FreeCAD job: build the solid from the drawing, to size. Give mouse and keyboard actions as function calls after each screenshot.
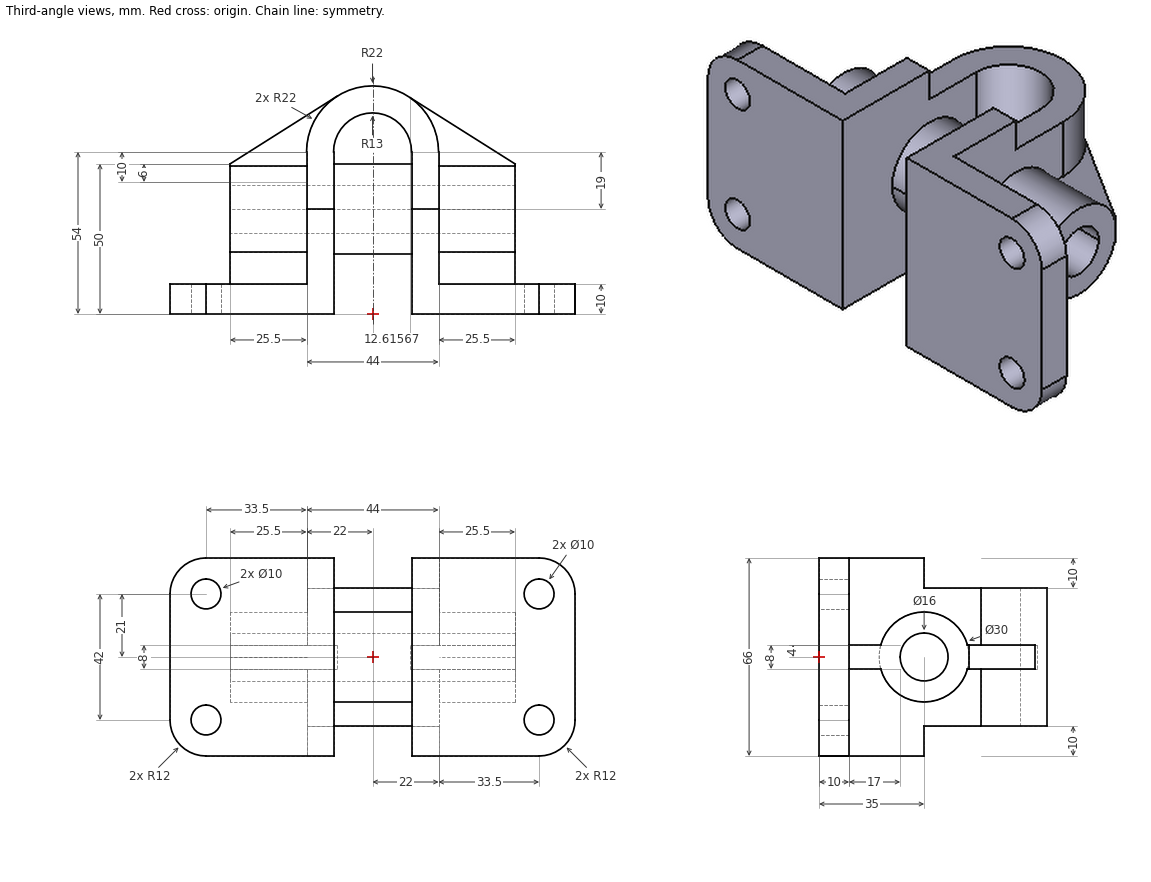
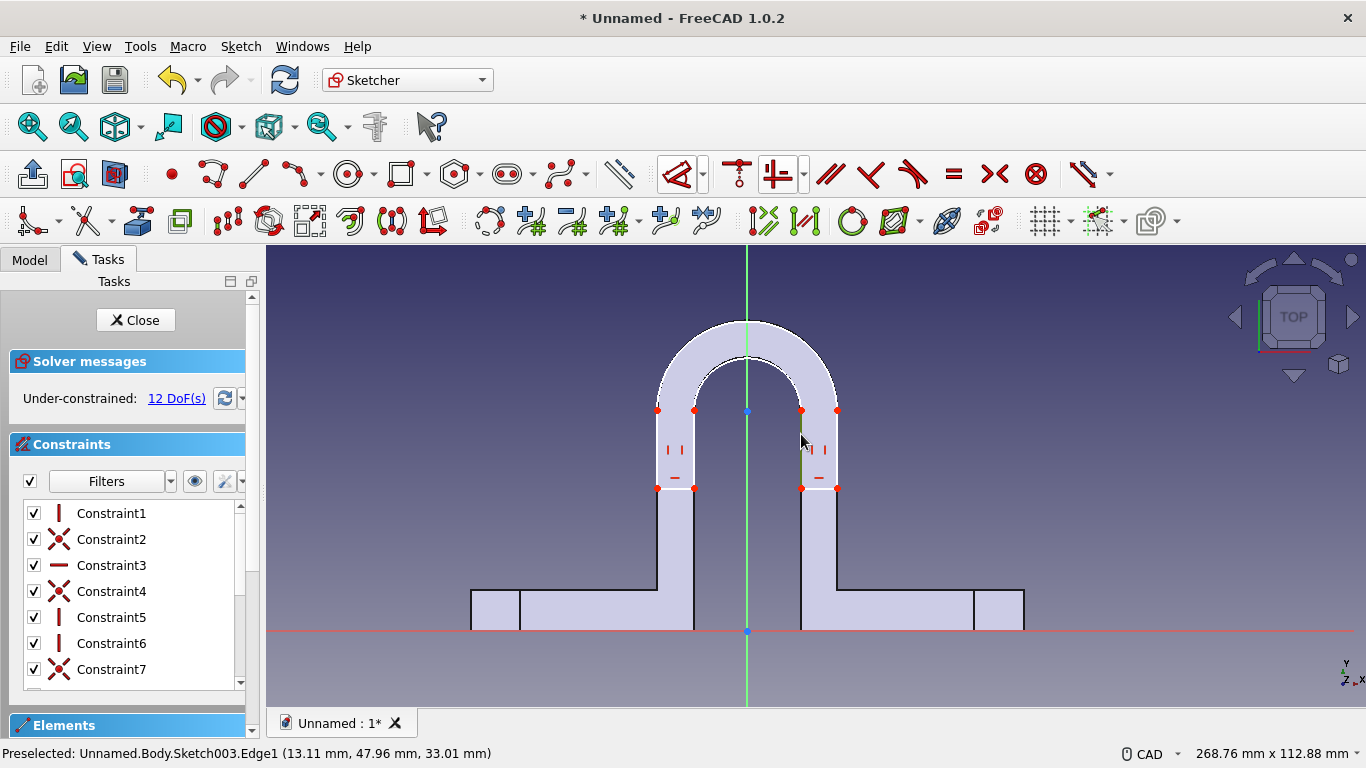
click(779, 368)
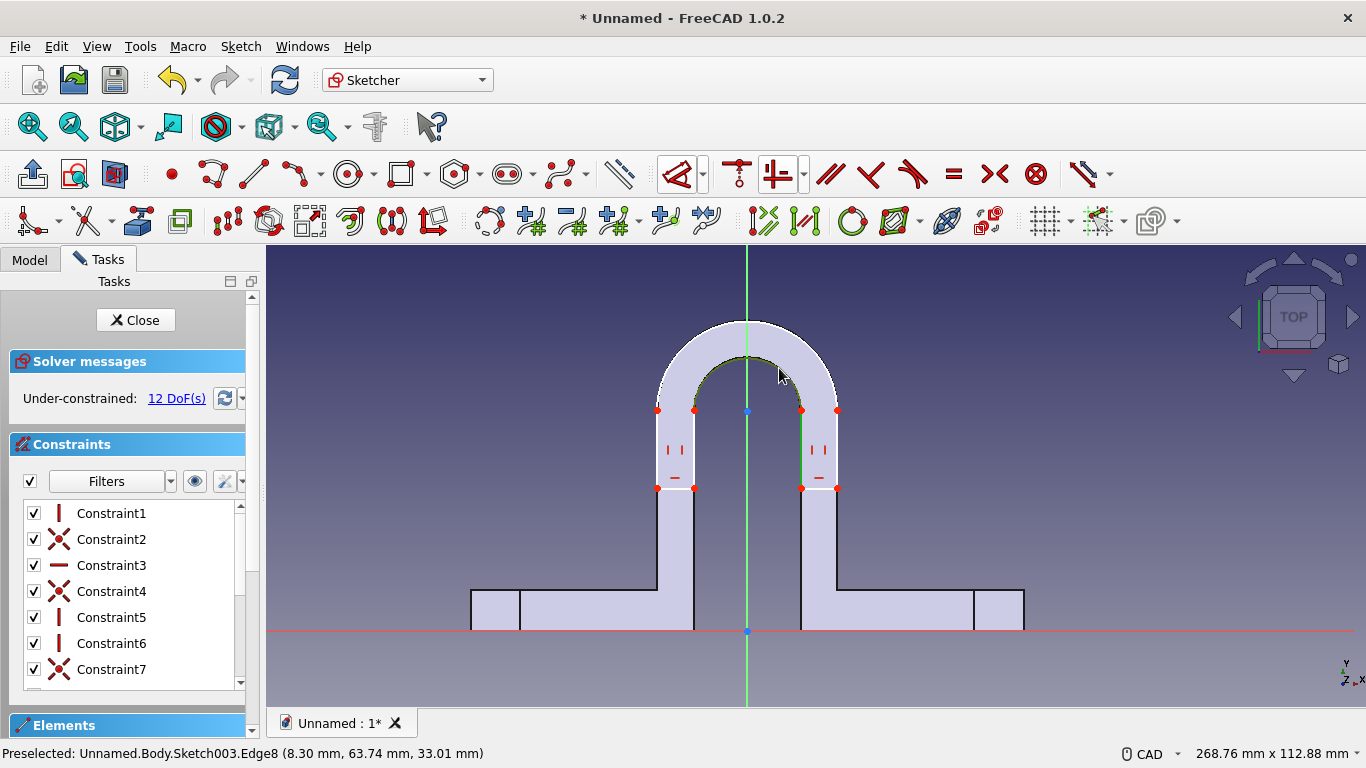
click(913, 174)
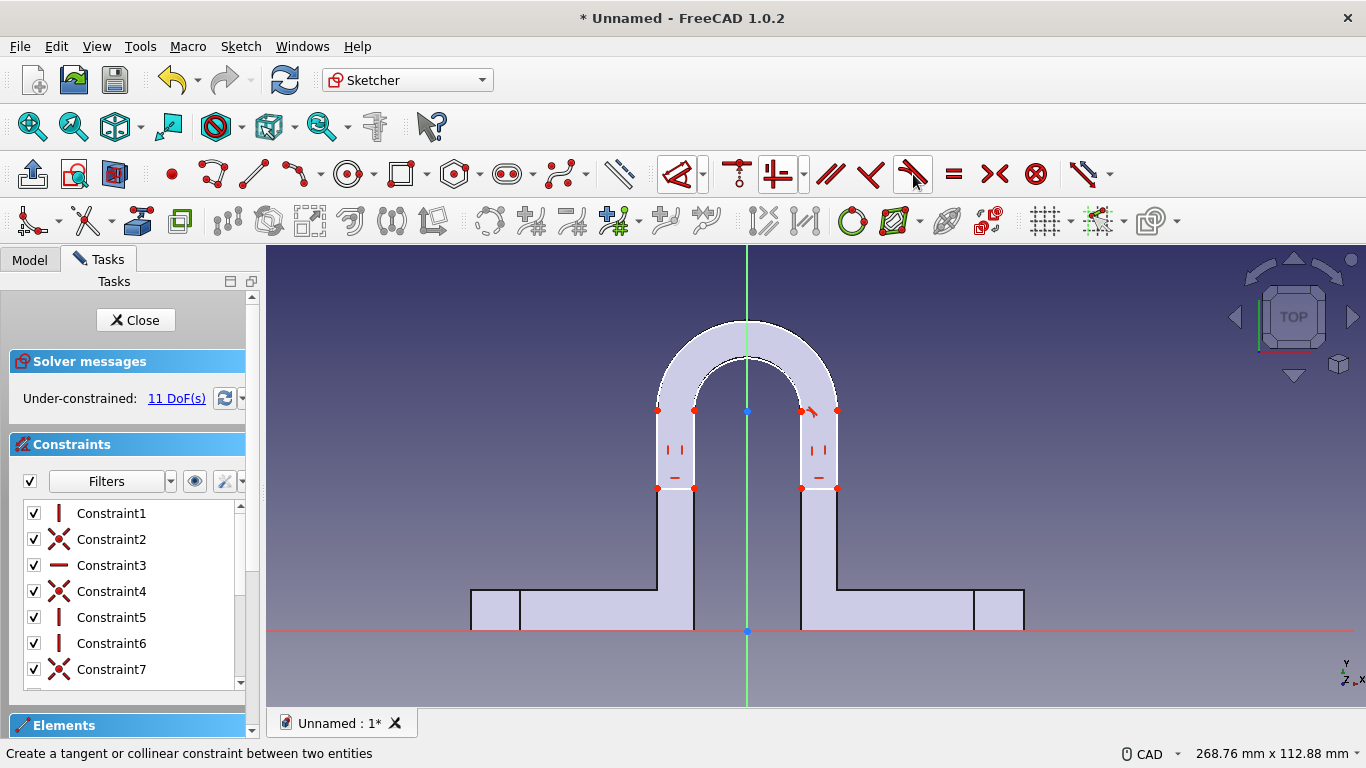
click(837, 466)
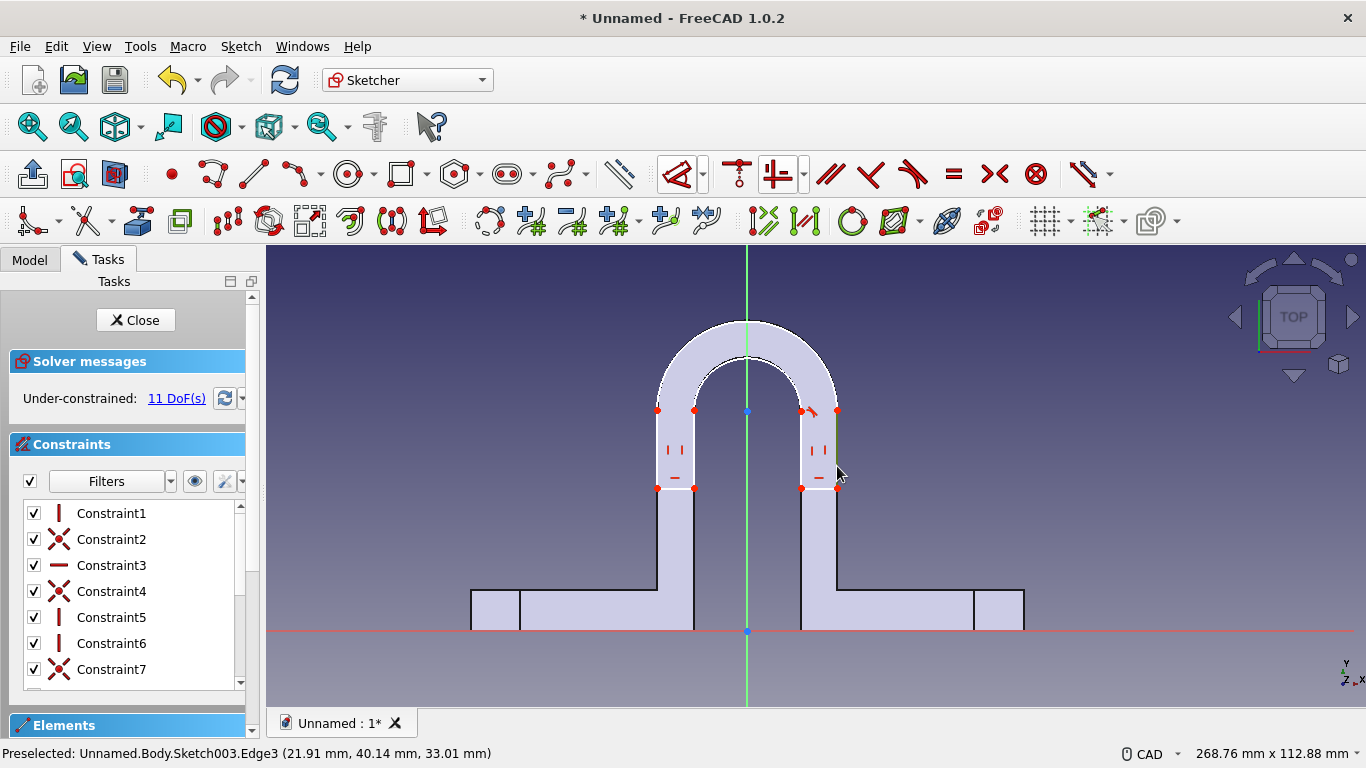
click(800, 339)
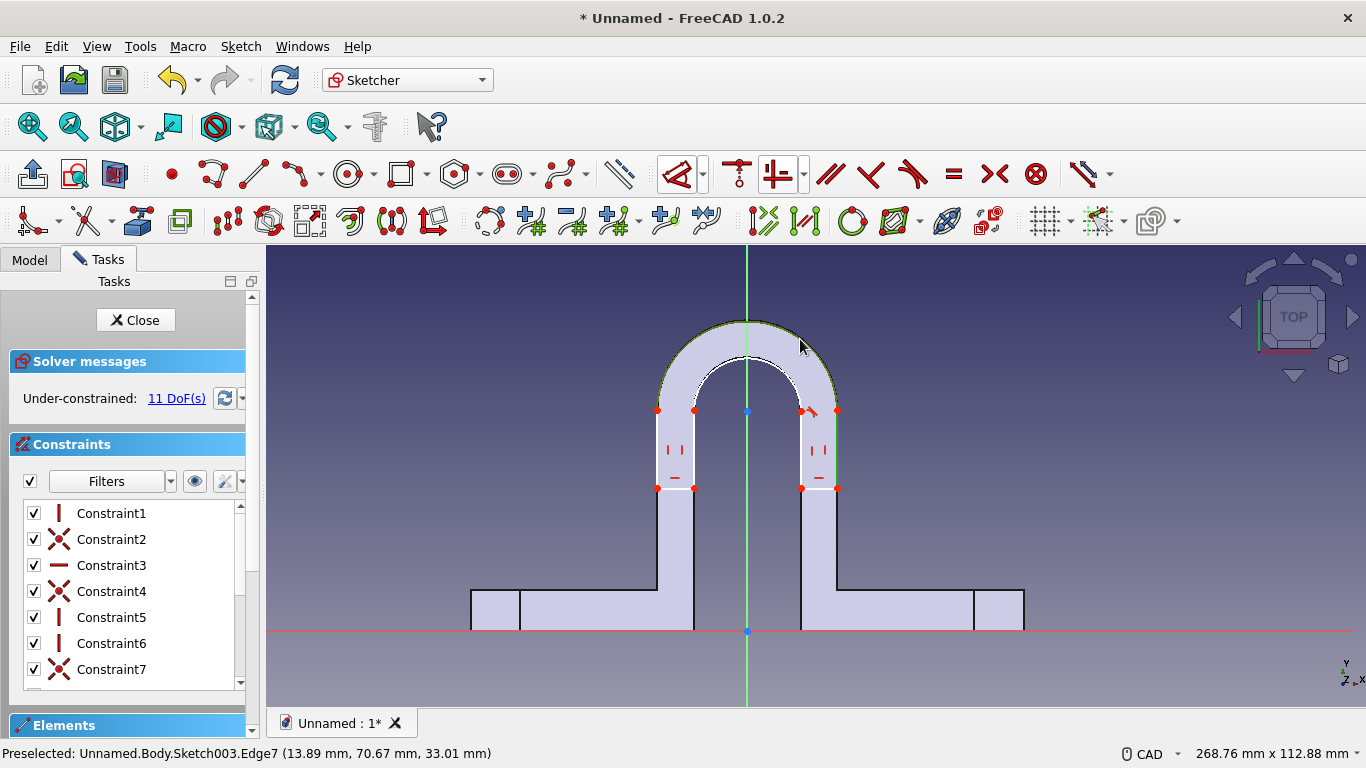
click(913, 174)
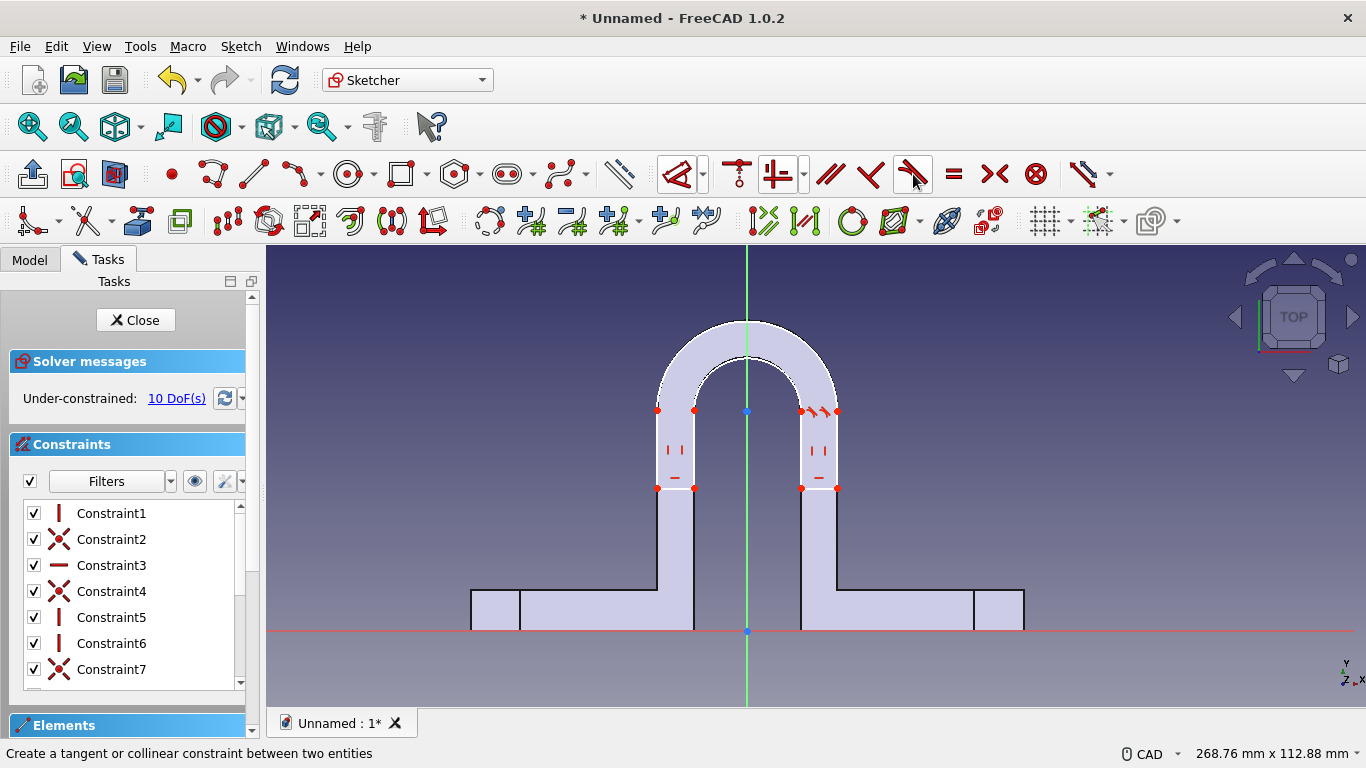
click(657, 434)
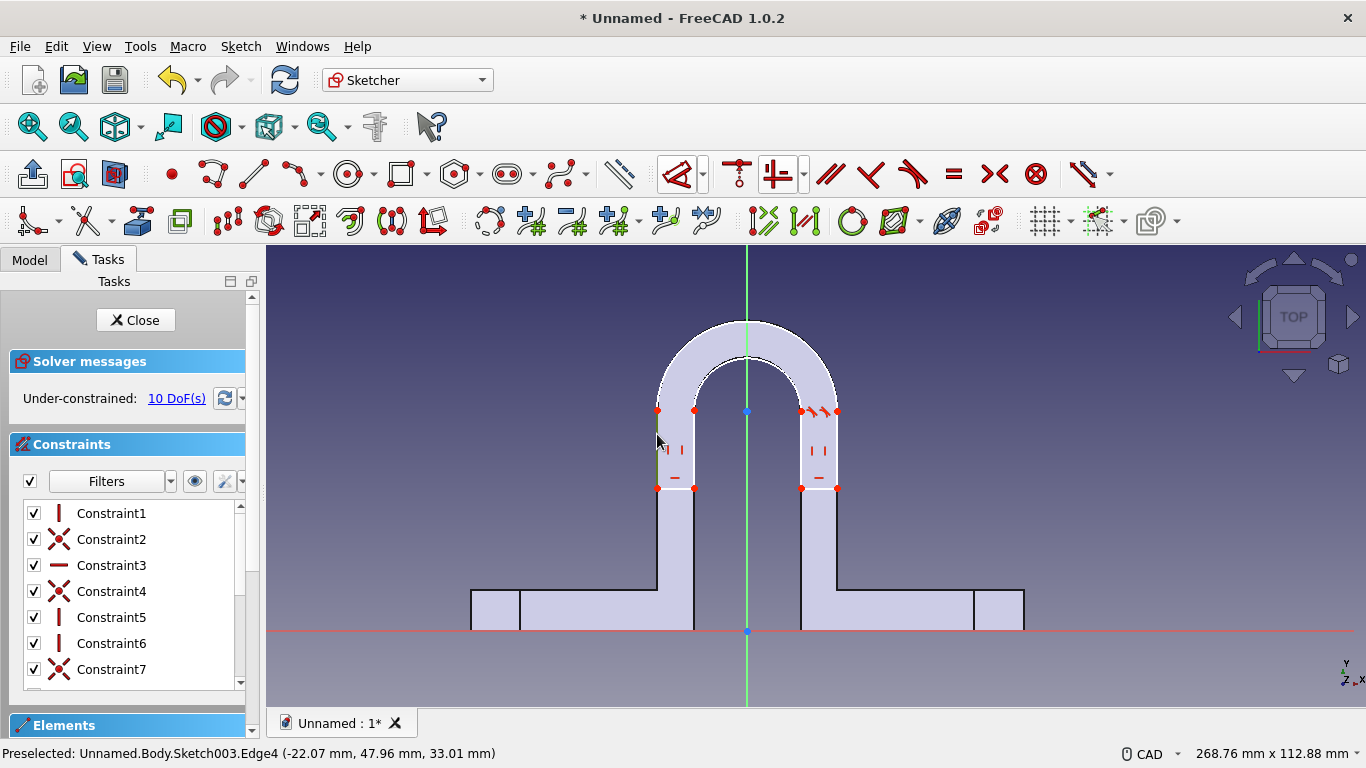
click(800, 339)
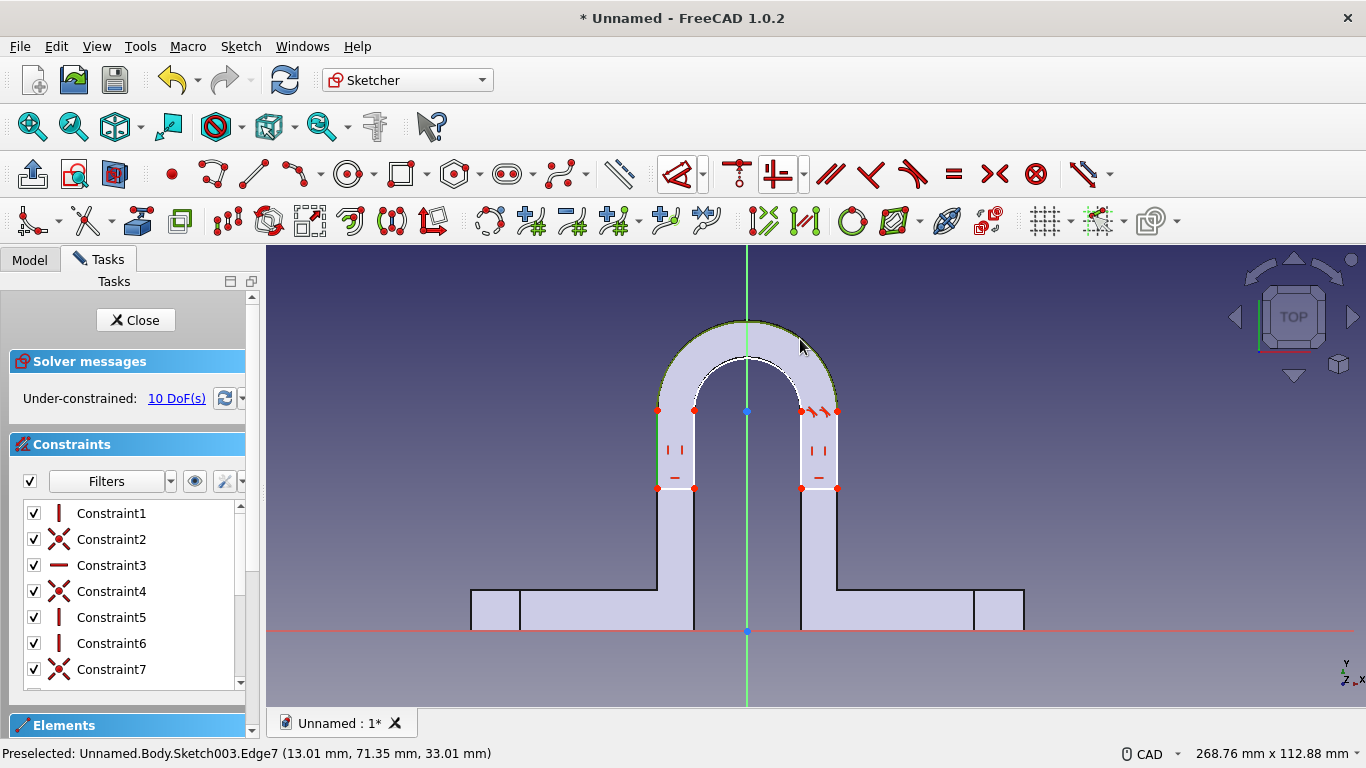
click(913, 174)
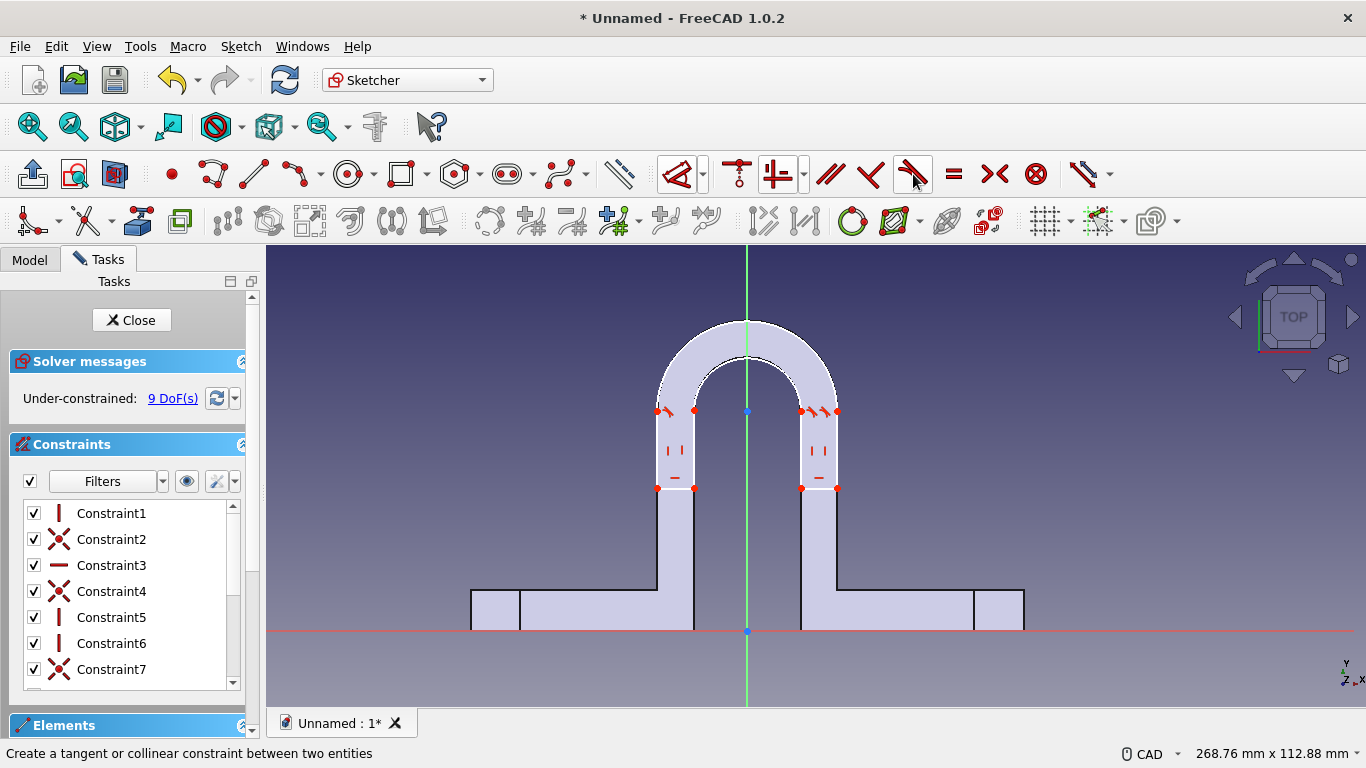
click(694, 466)